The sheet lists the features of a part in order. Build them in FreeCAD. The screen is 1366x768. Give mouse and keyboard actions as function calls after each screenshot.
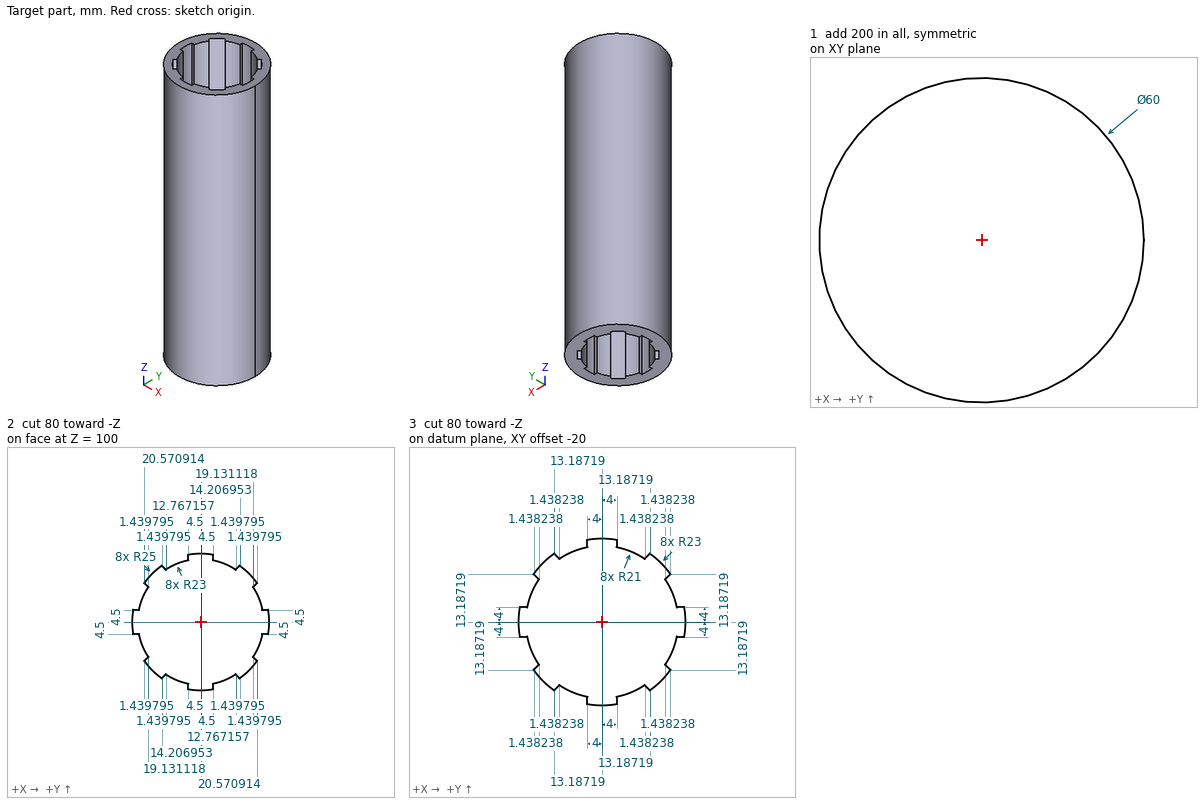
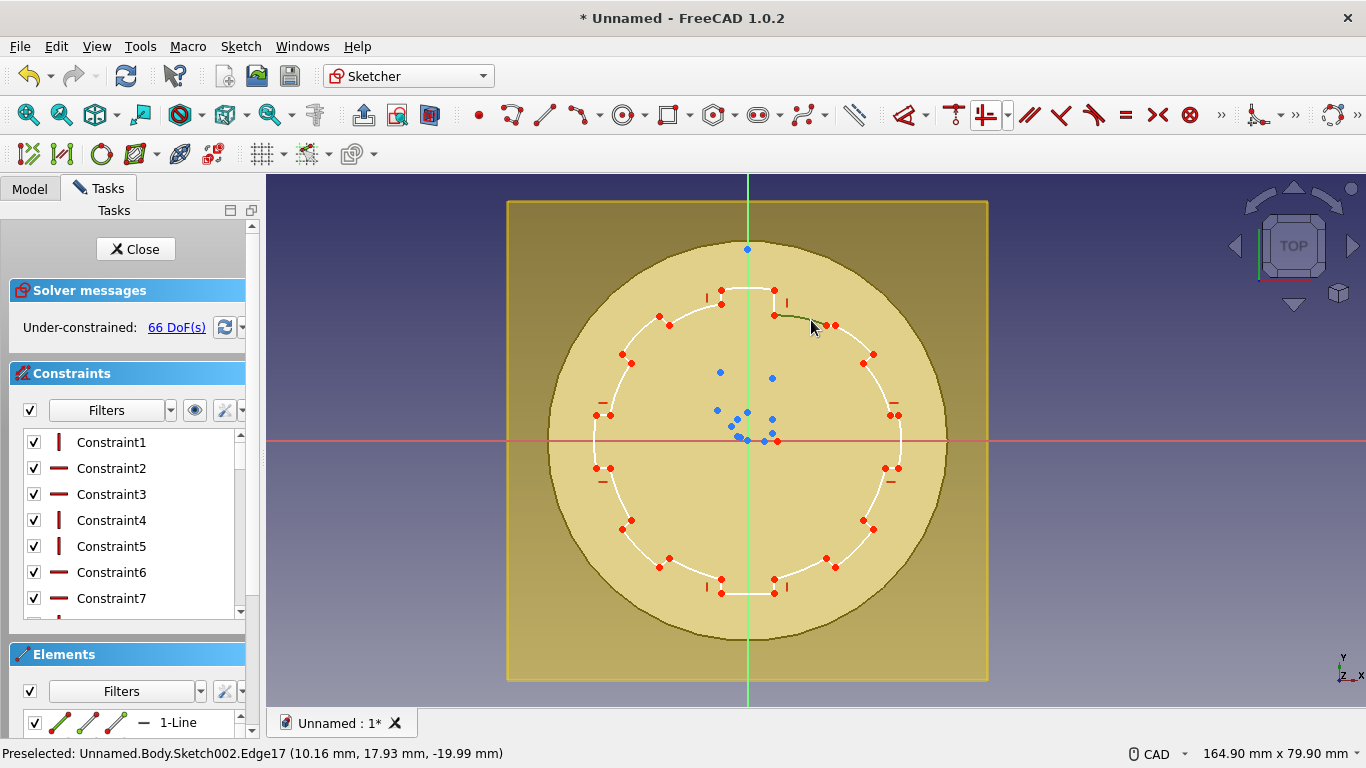
click(872, 506)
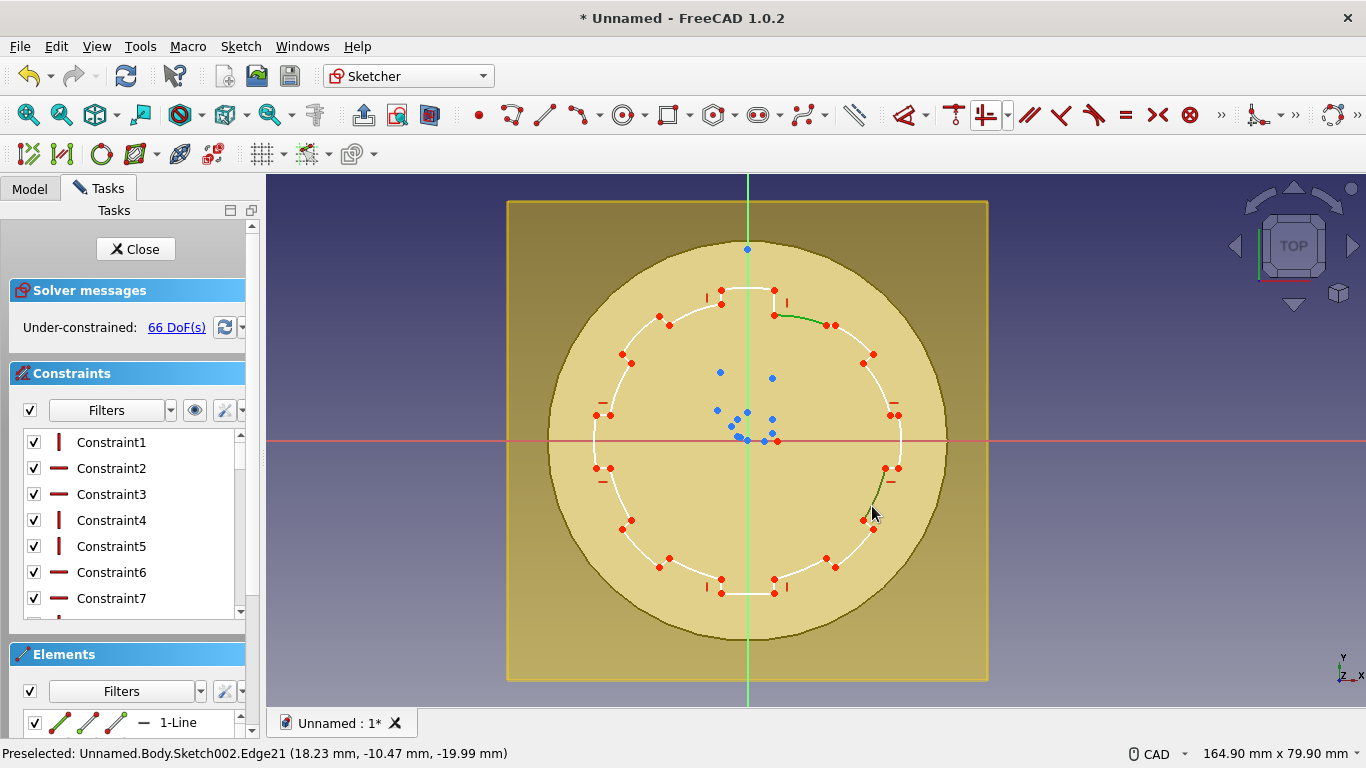
click(954, 116)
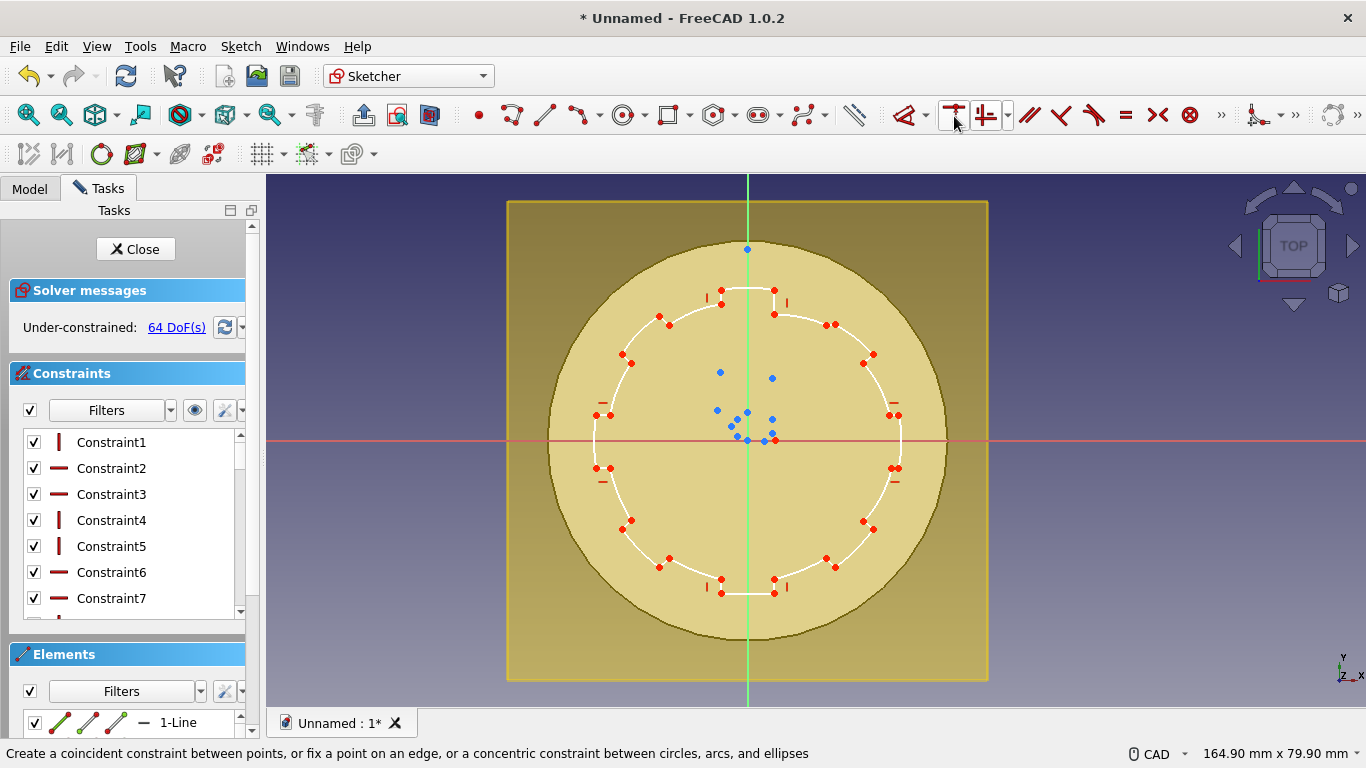
click(811, 320)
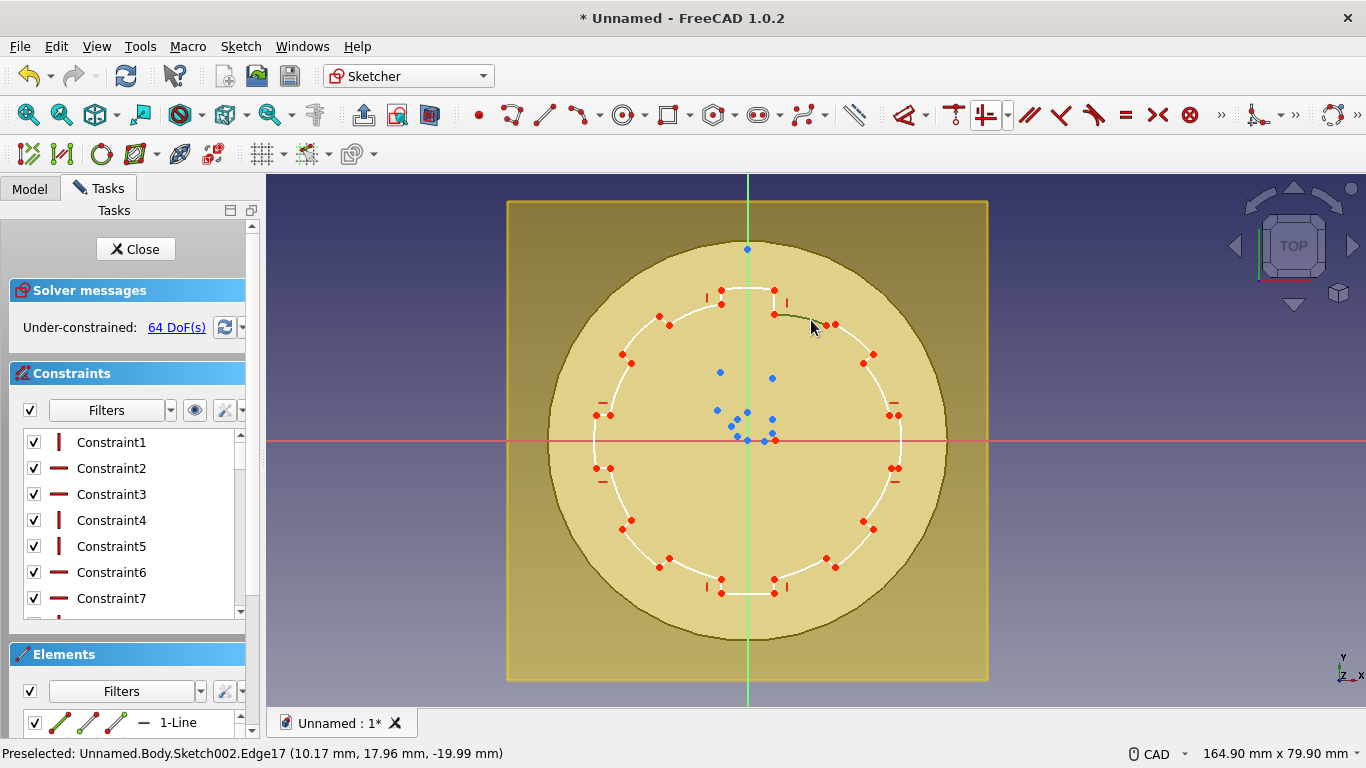
click(848, 557)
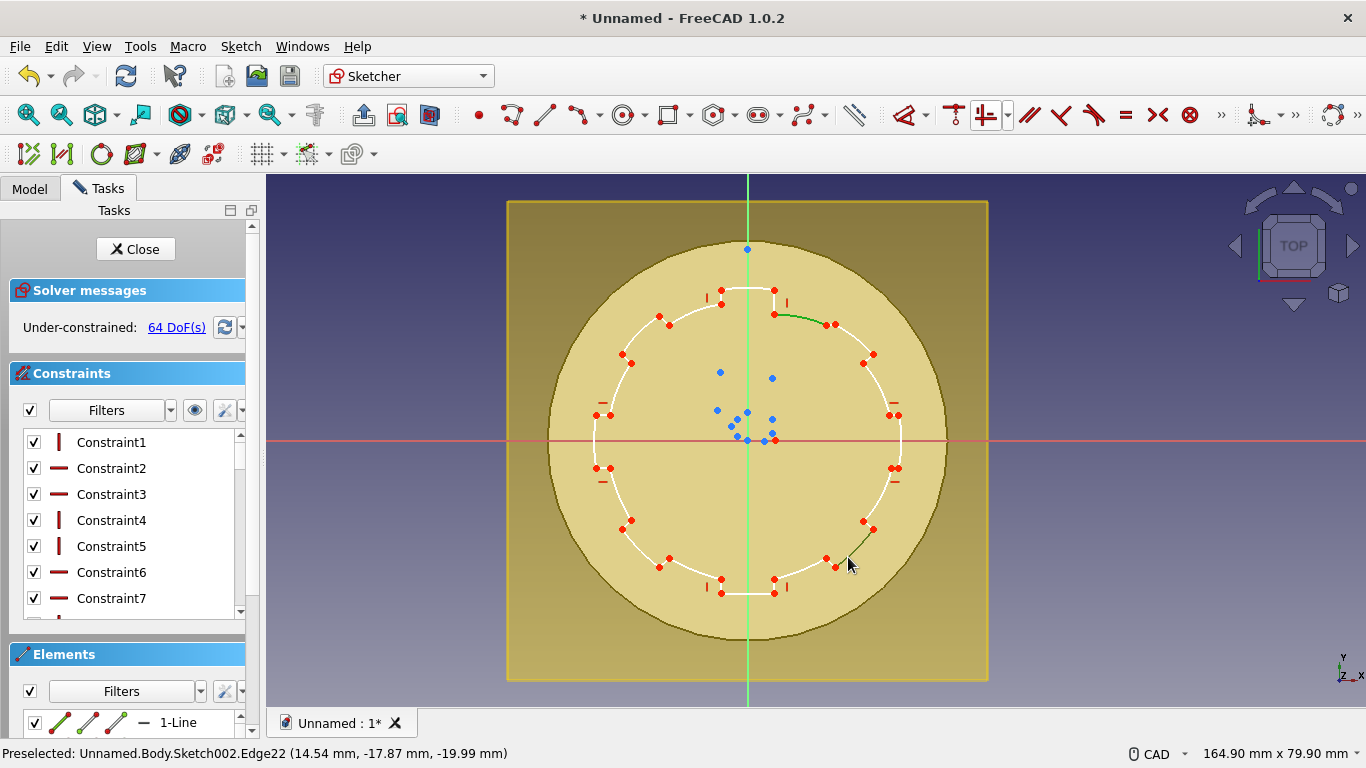
click(954, 116)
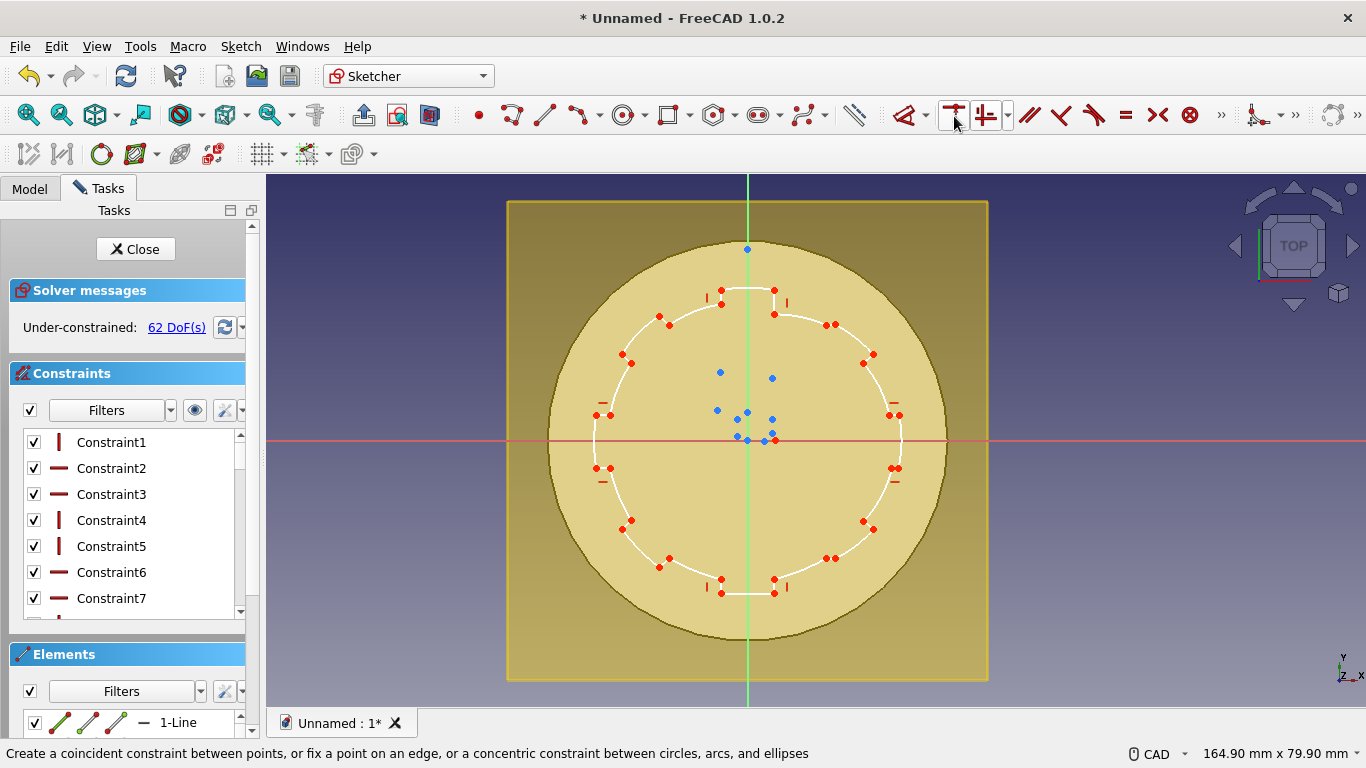
click(811, 320)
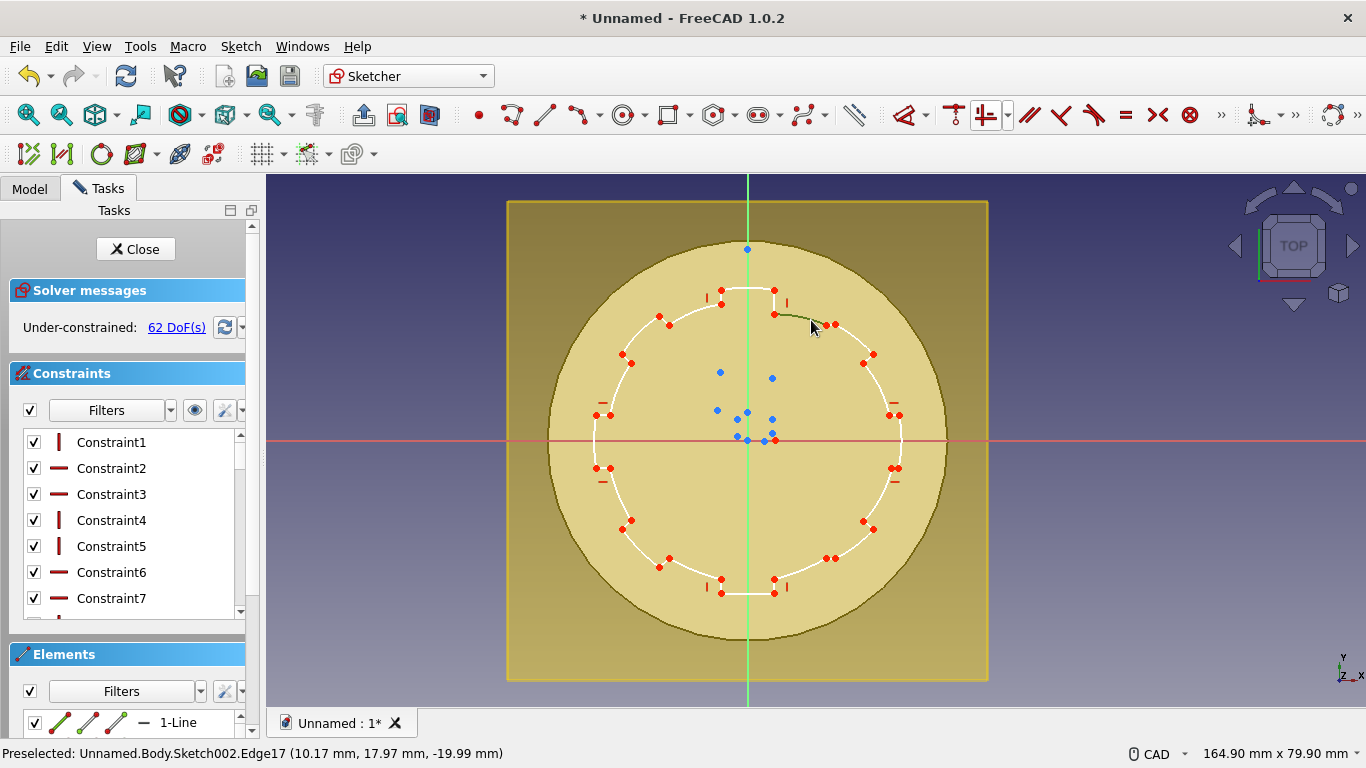
click(790, 575)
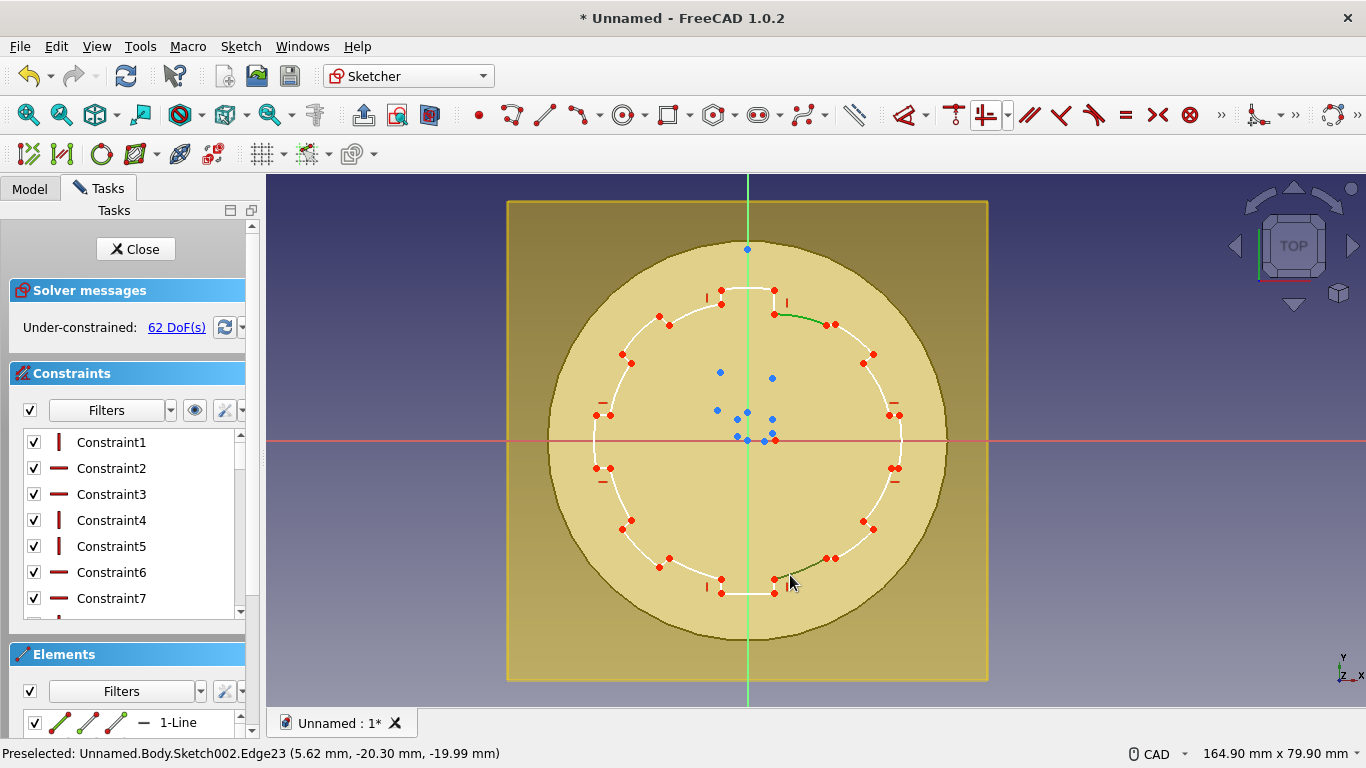
click(954, 116)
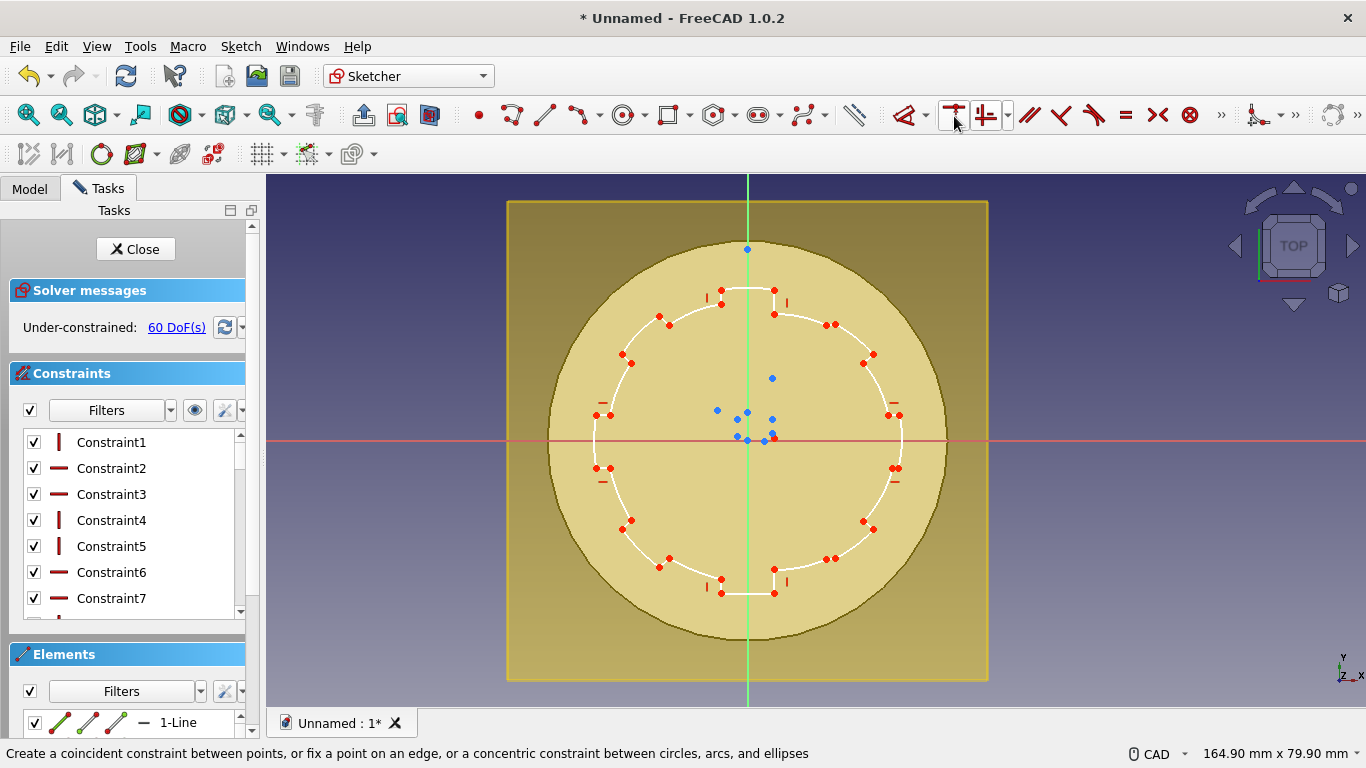
click(811, 320)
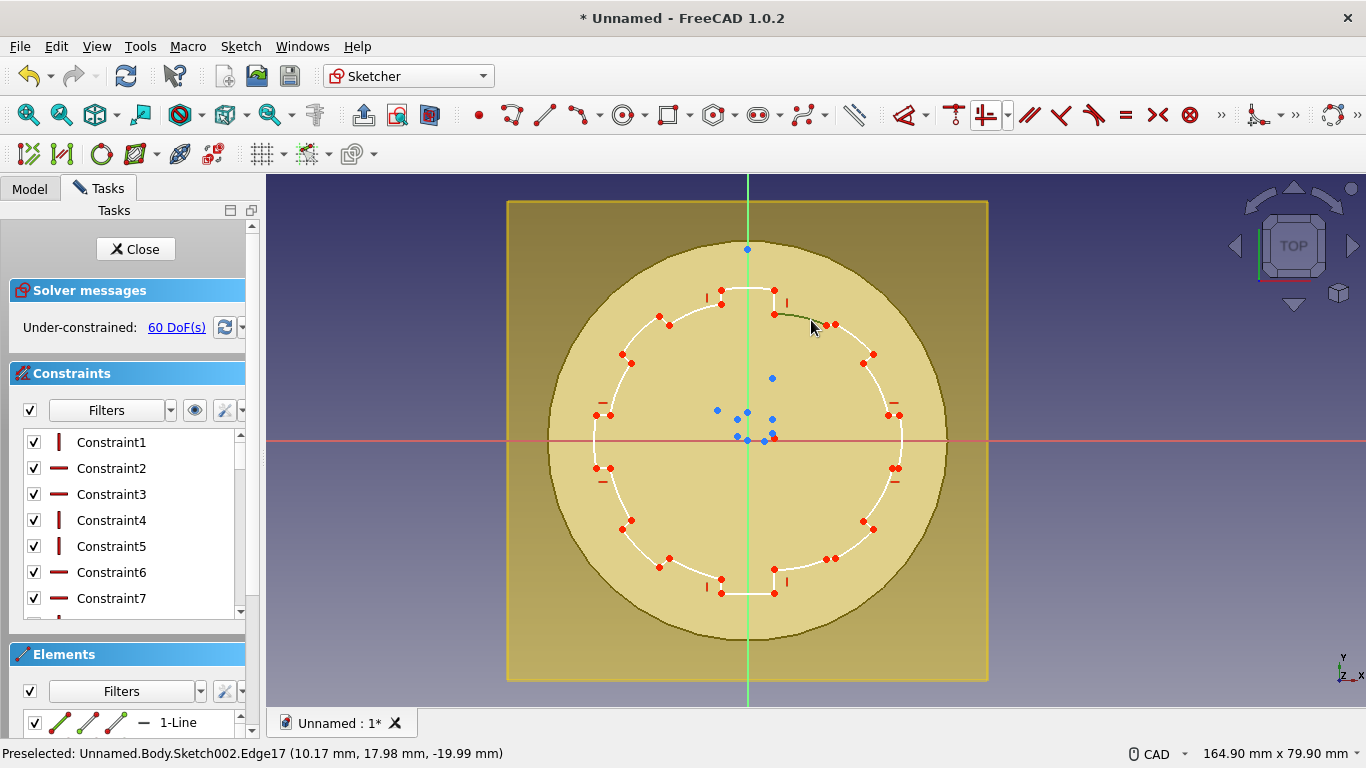
scroll(737, 594, up, 2)